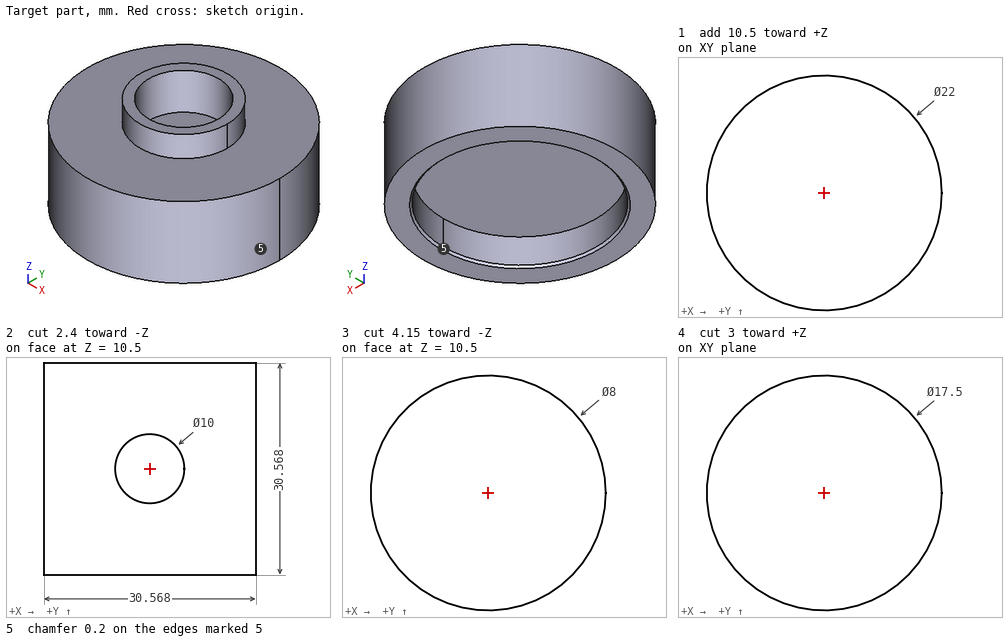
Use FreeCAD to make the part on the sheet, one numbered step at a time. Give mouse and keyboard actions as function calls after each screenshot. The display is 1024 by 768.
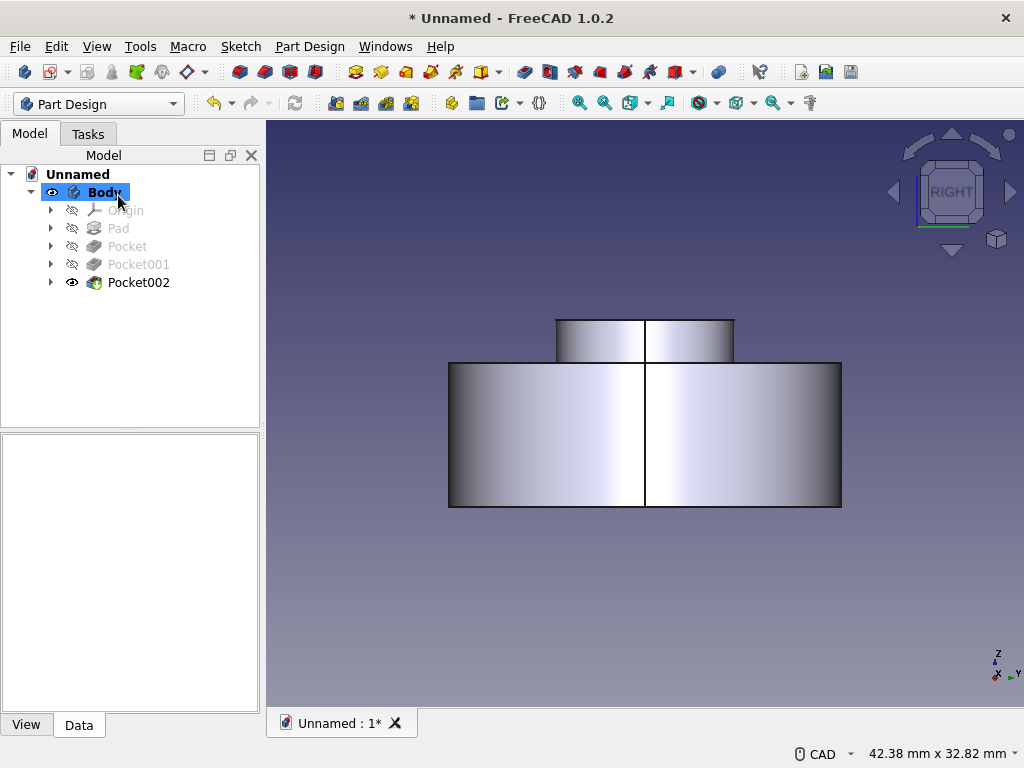
key(5)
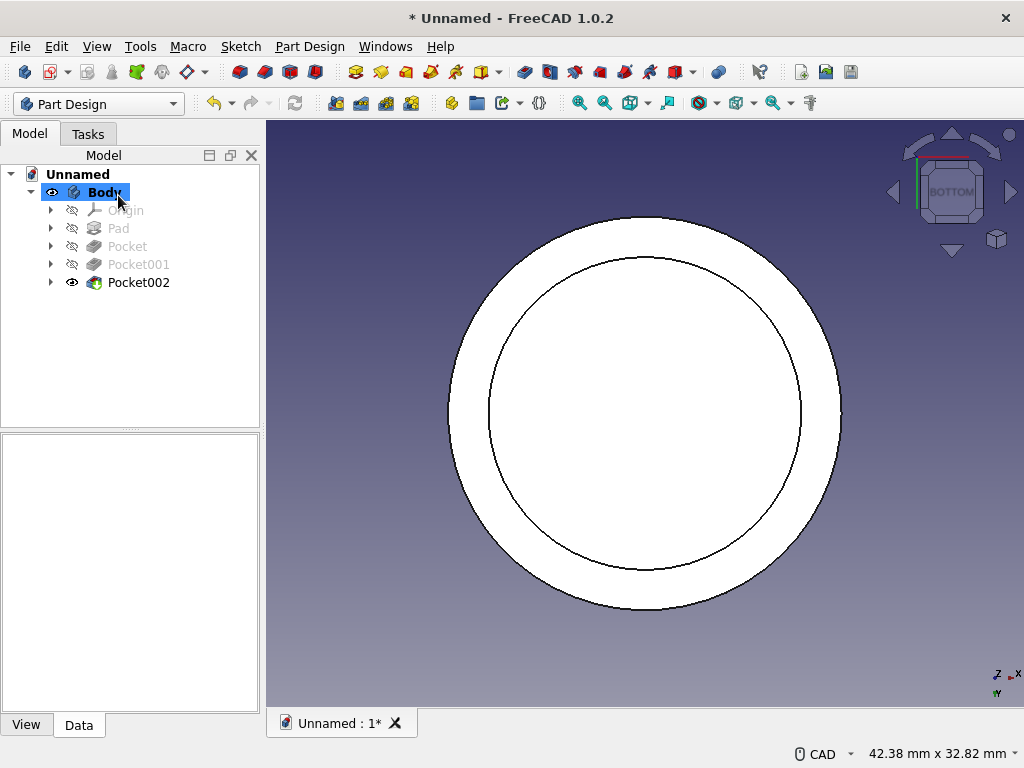
click(488, 413)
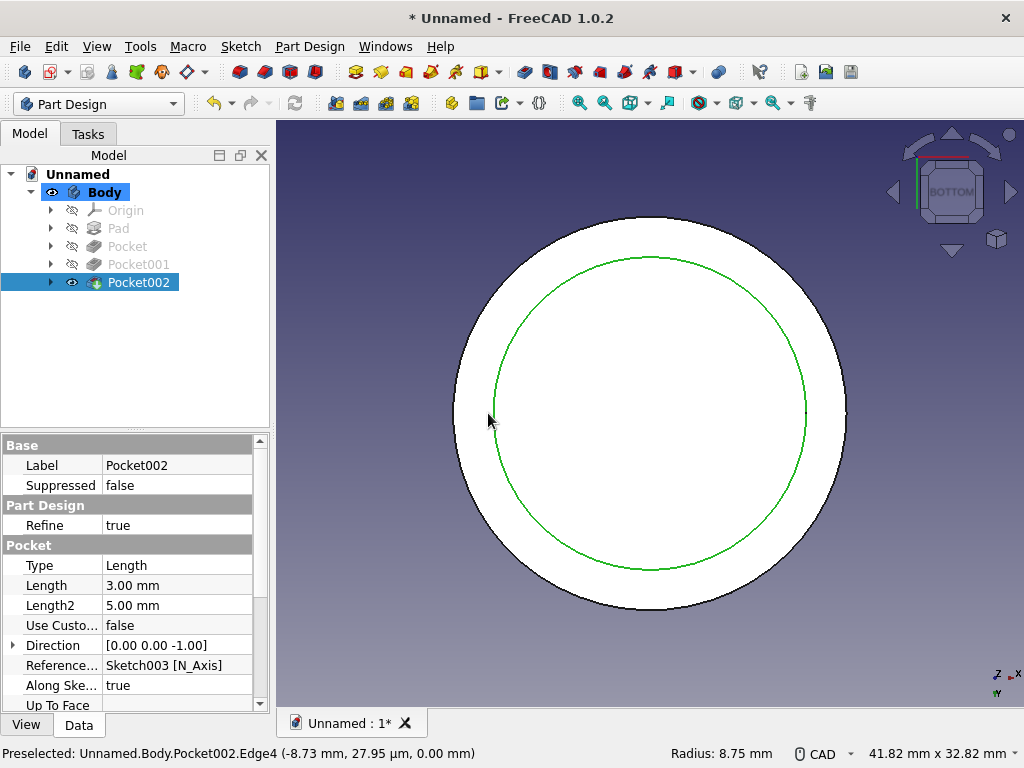
click(265, 72)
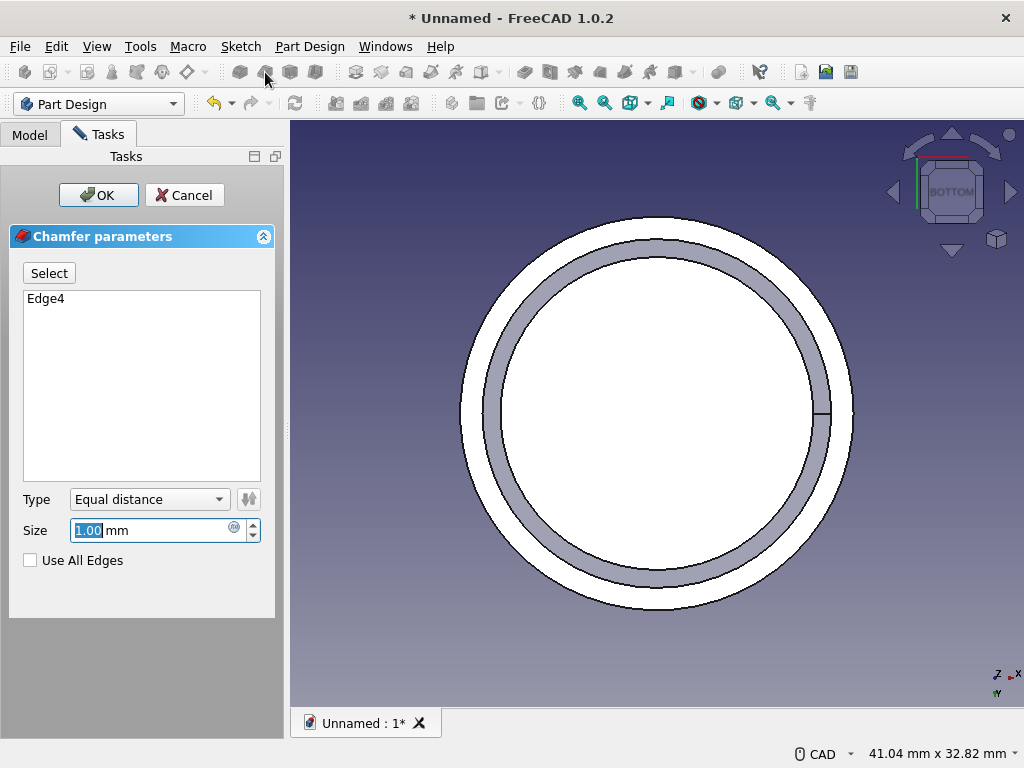
text(0.2)
key(Tab)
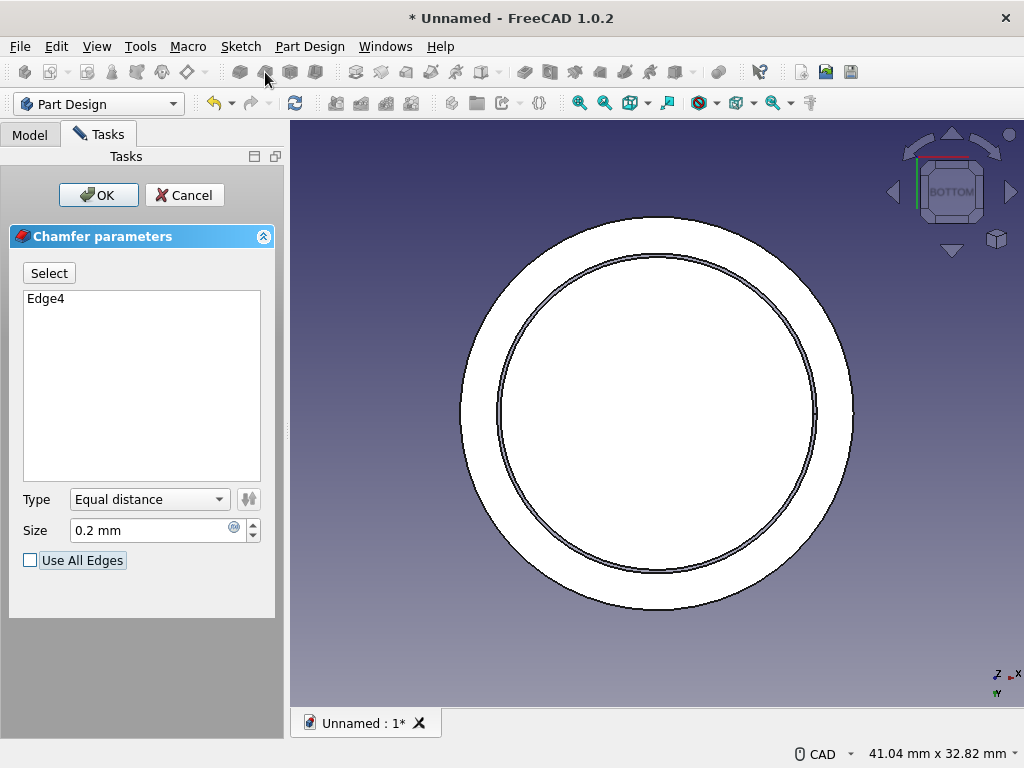
click(99, 195)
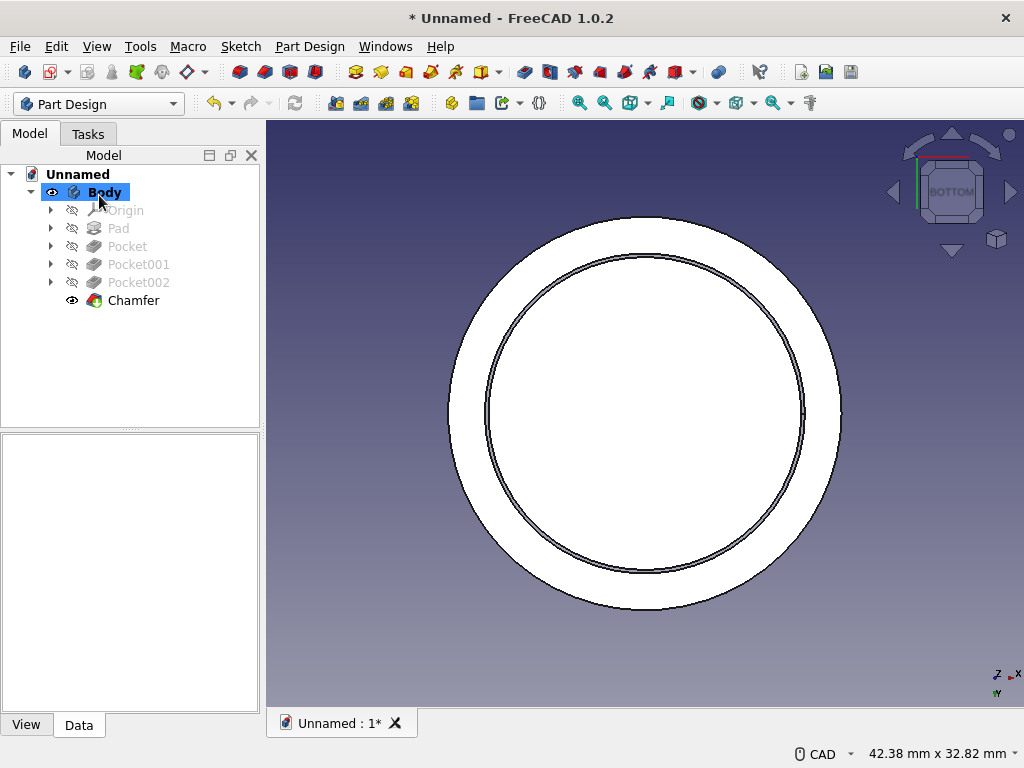
key(0)